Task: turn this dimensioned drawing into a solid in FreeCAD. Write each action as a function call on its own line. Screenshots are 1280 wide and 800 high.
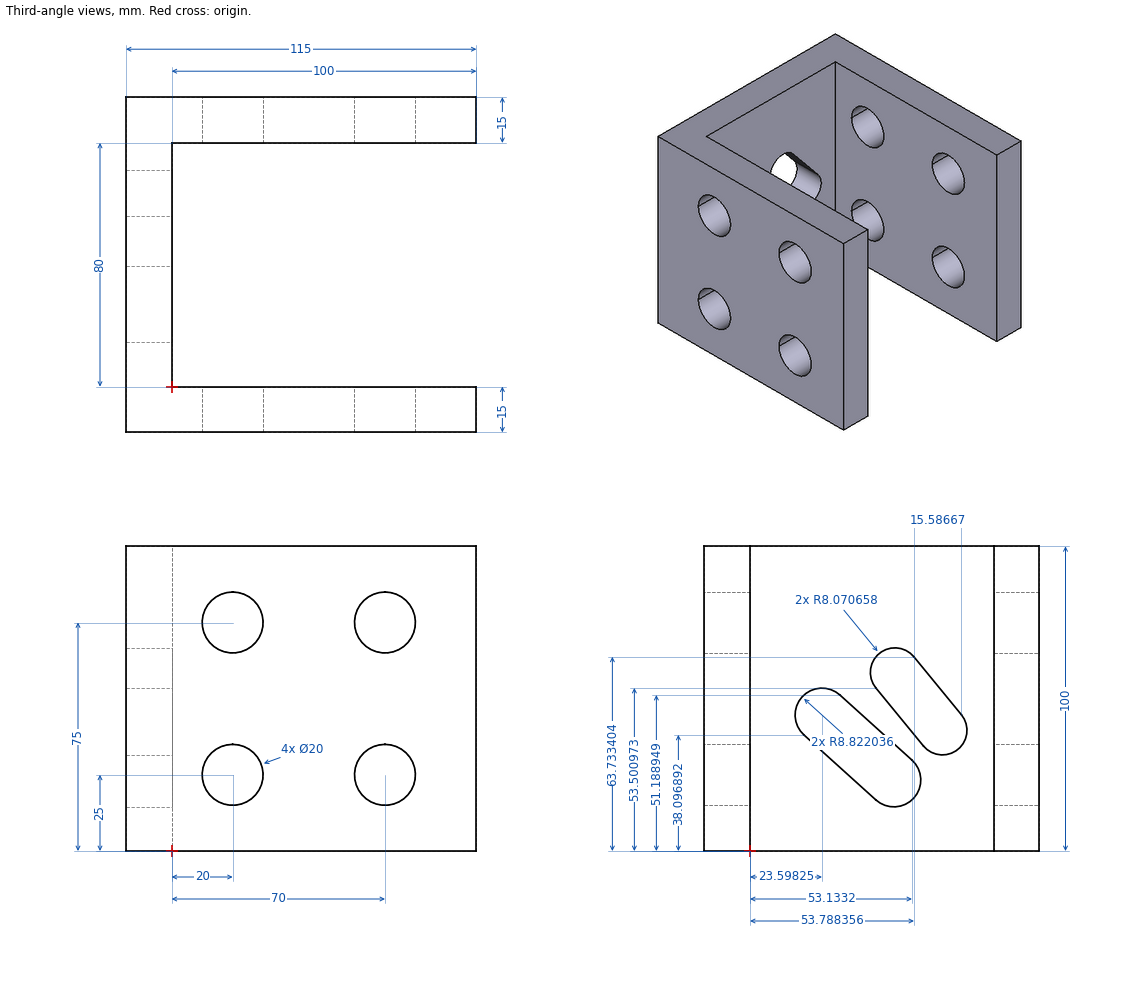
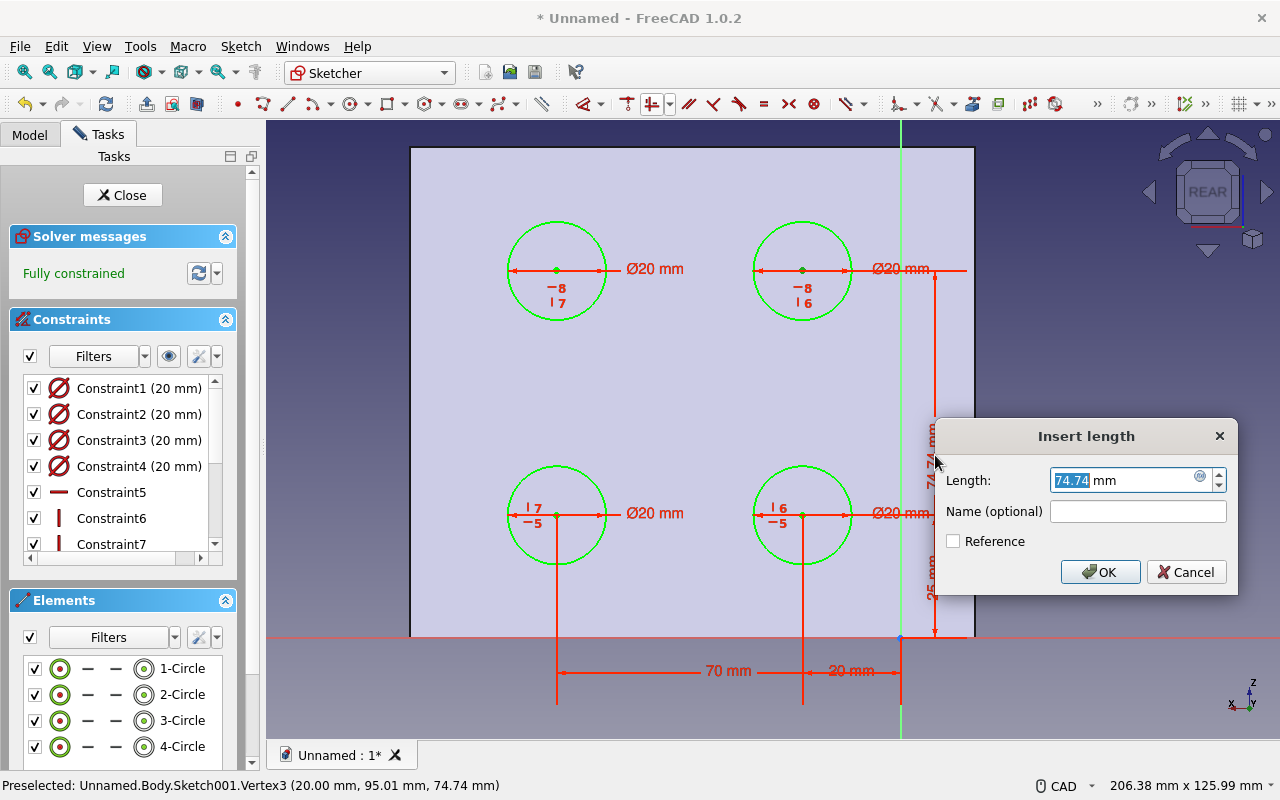
text(75)
key(Return)
key(Escape)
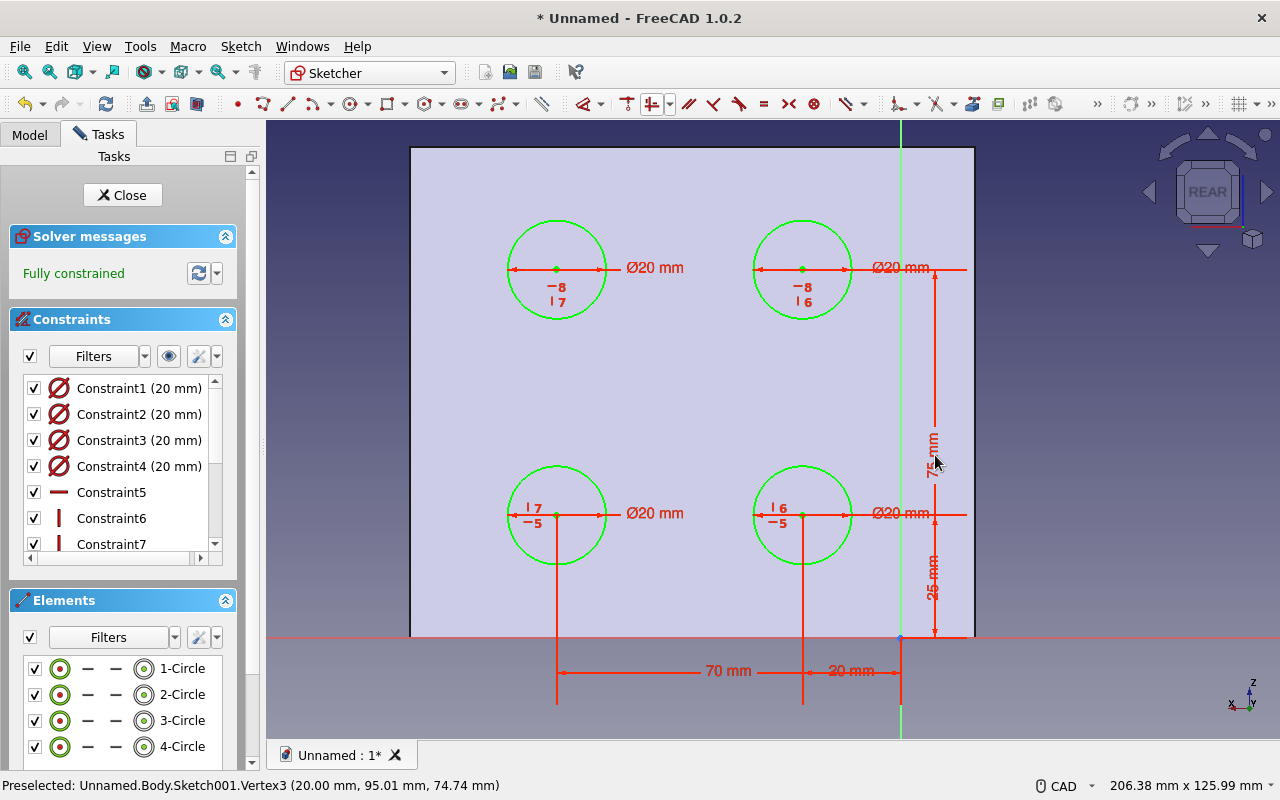
click(123, 195)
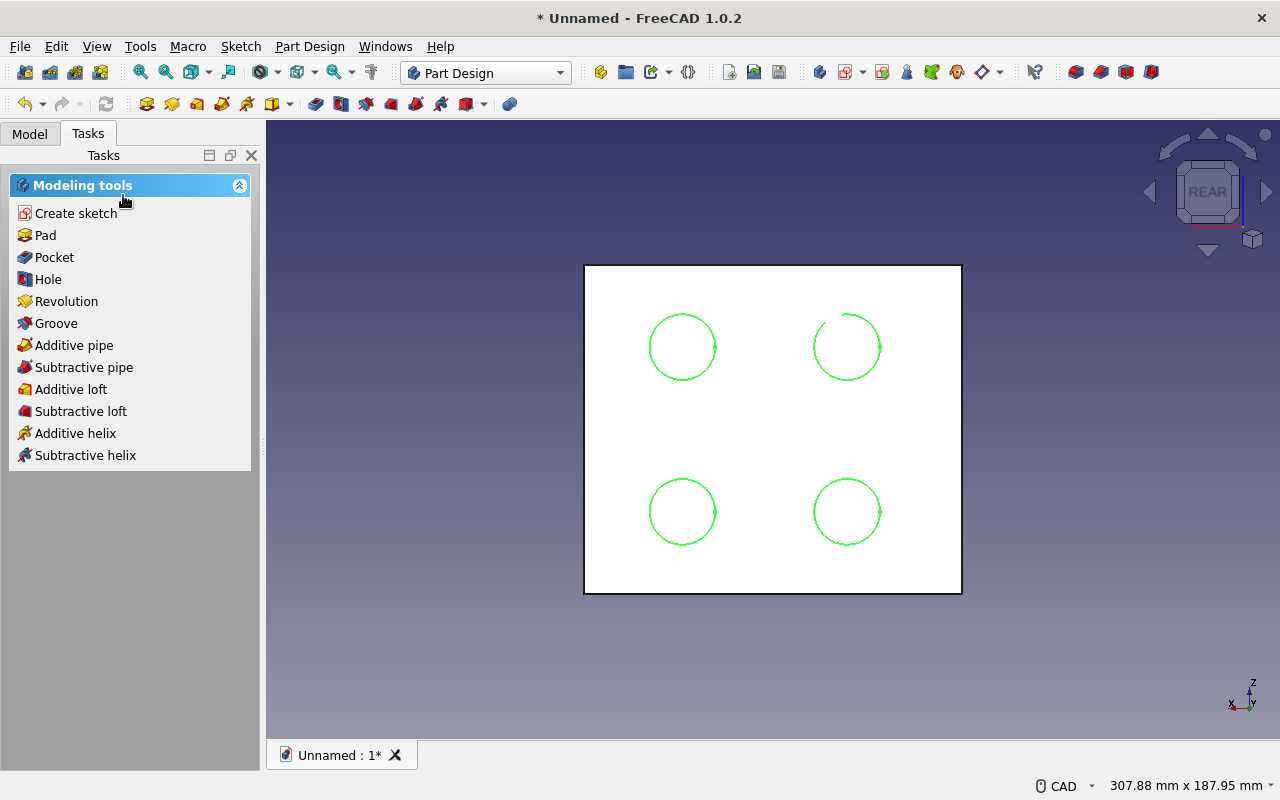
click(316, 104)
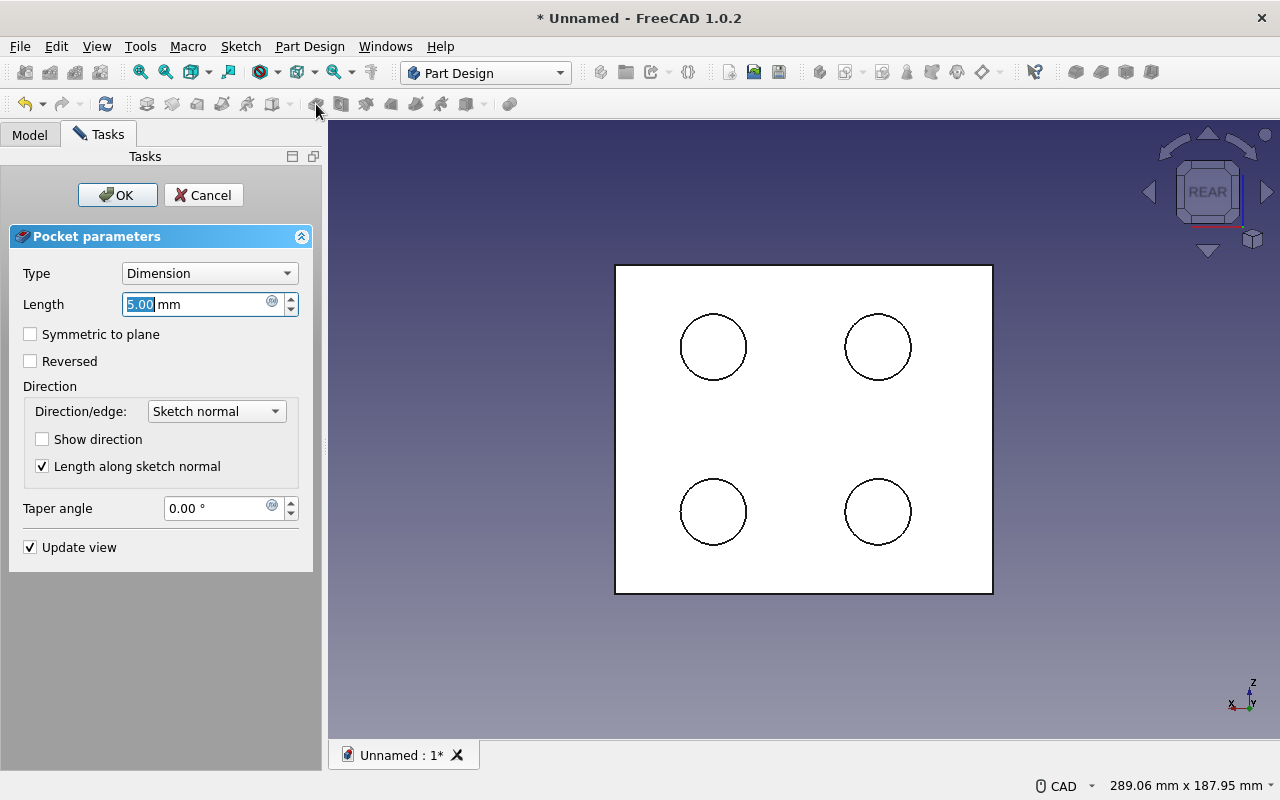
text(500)
key(Tab)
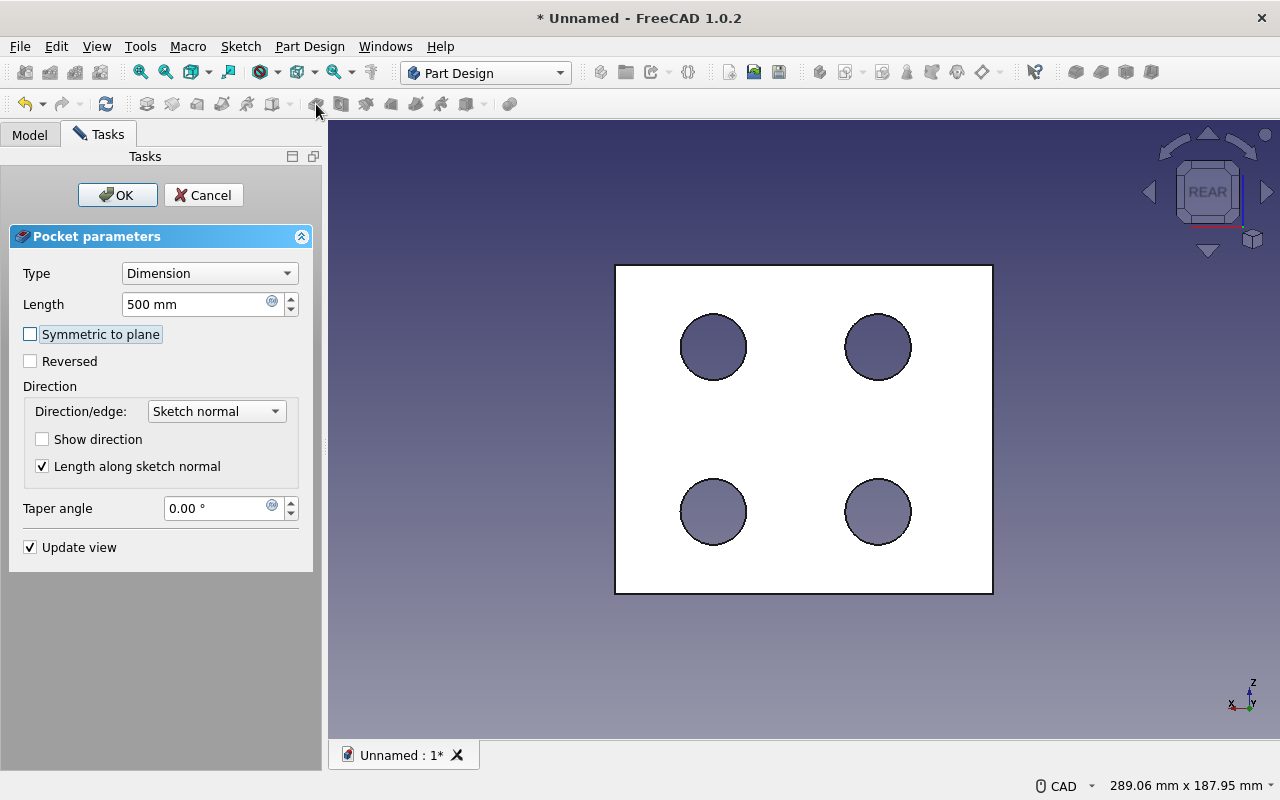
click(118, 195)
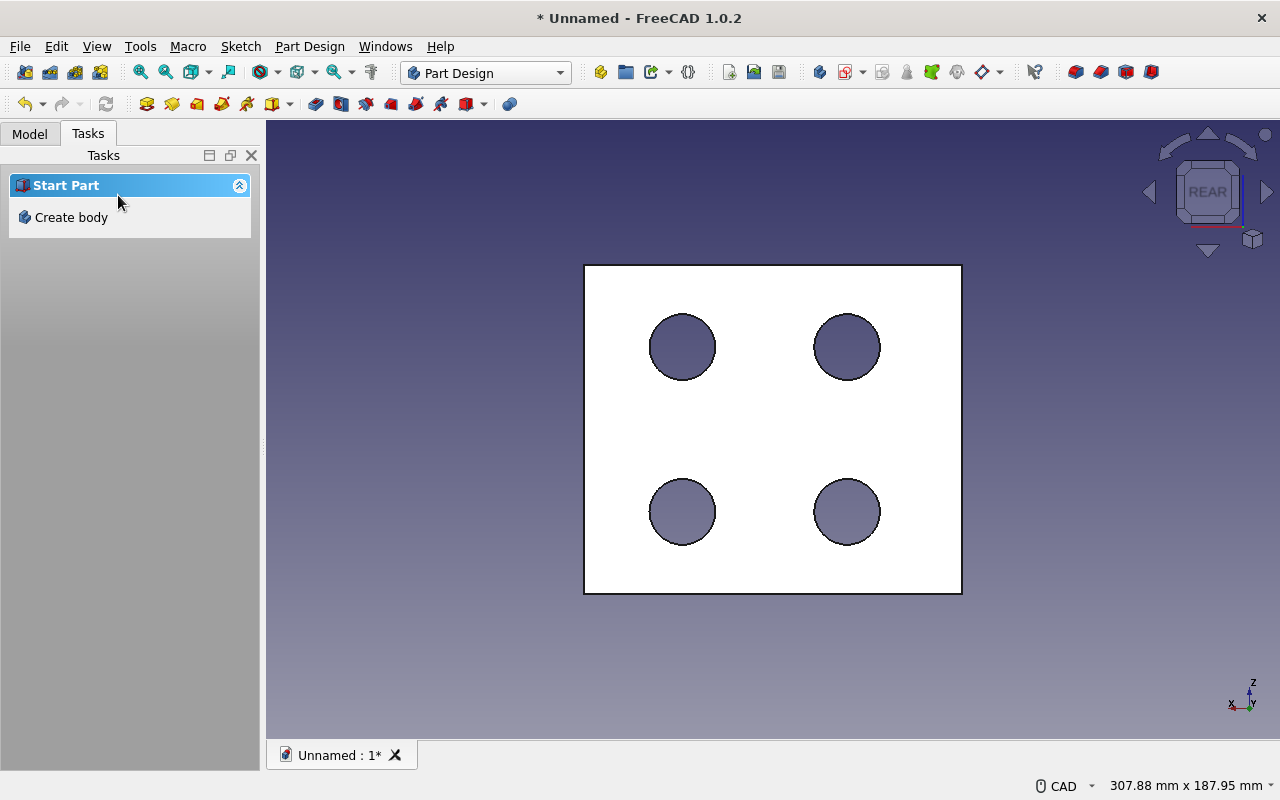
click(844, 72)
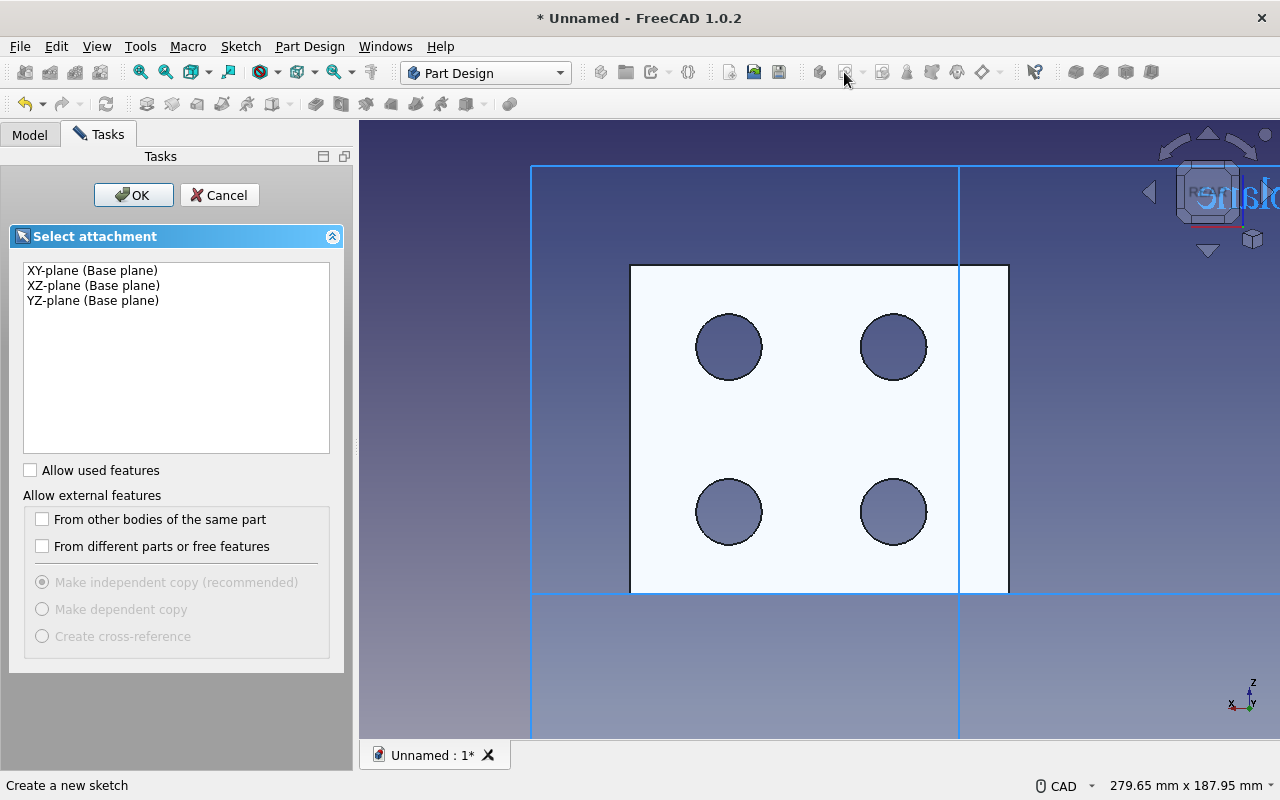
click(84, 300)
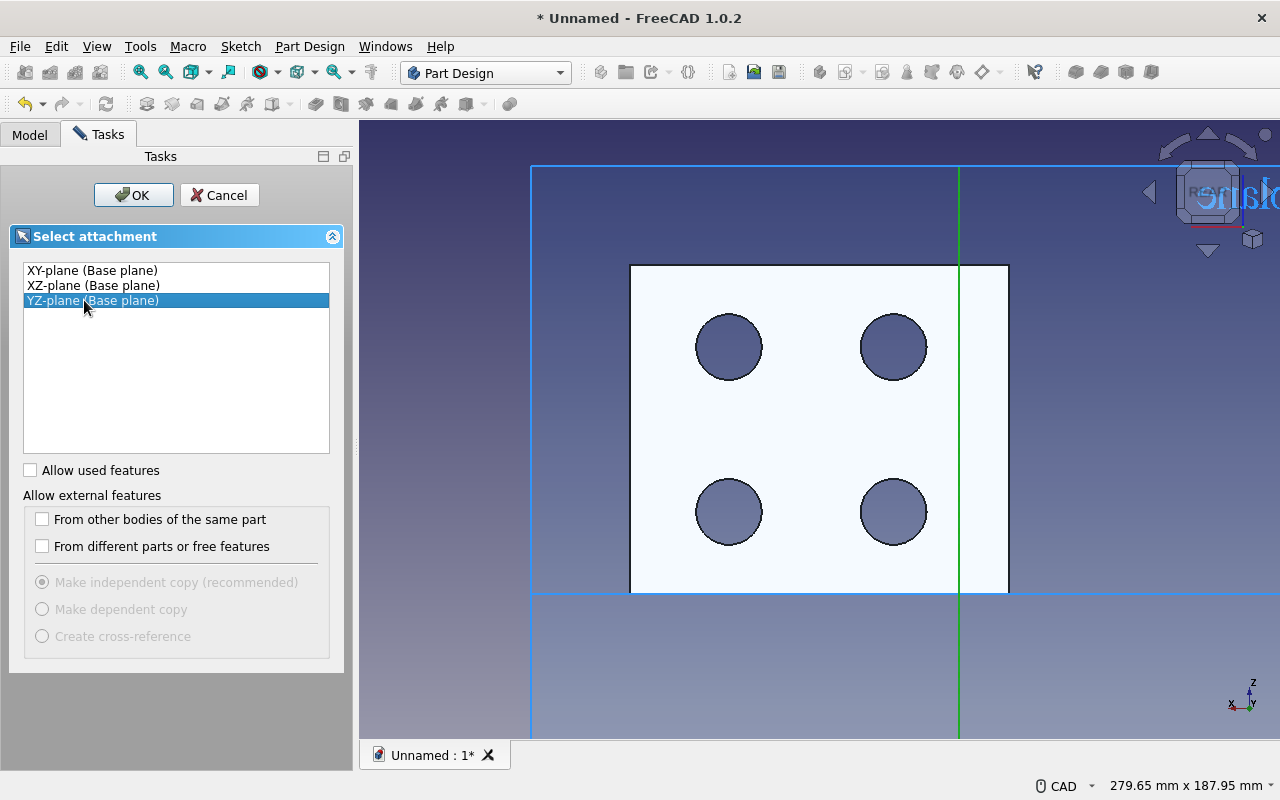
click(134, 195)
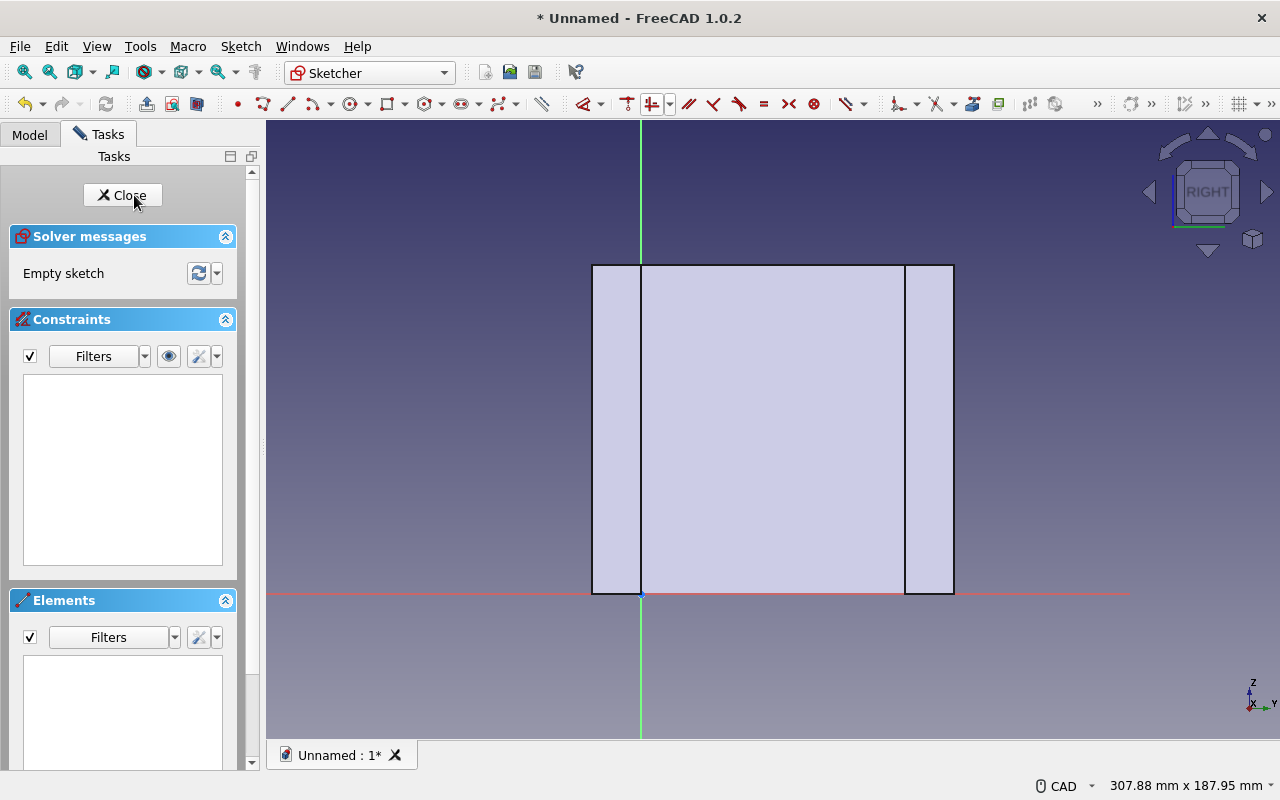
click(197, 104)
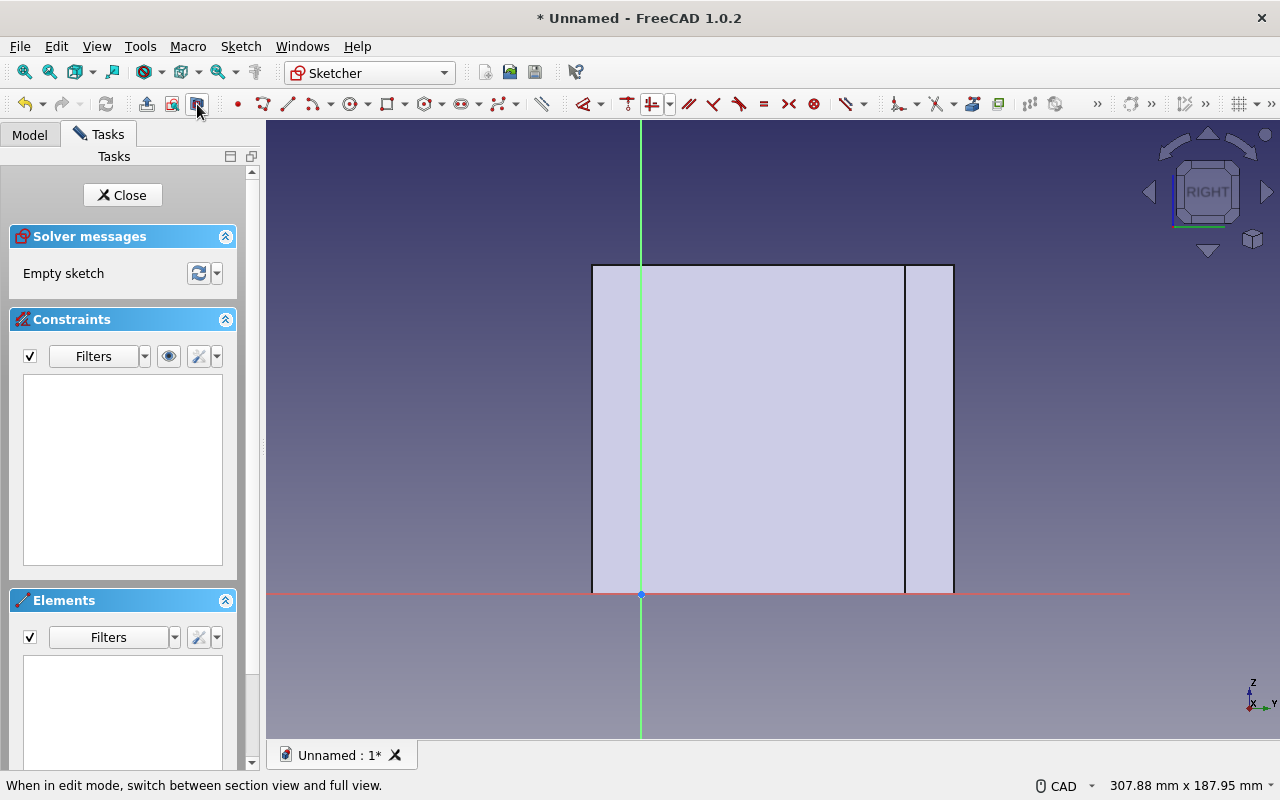
scroll(818, 558, up, 3)